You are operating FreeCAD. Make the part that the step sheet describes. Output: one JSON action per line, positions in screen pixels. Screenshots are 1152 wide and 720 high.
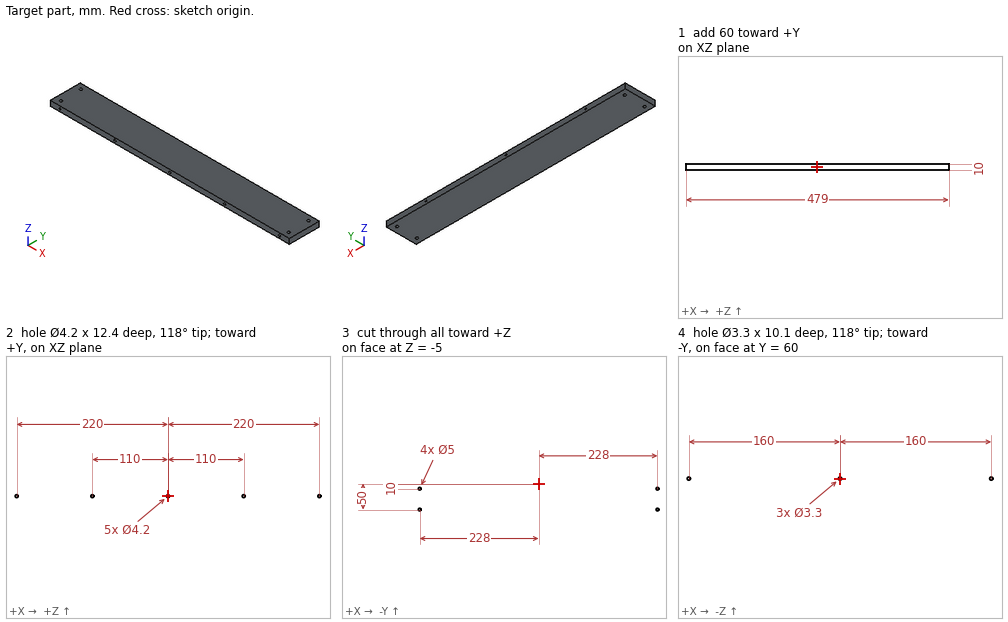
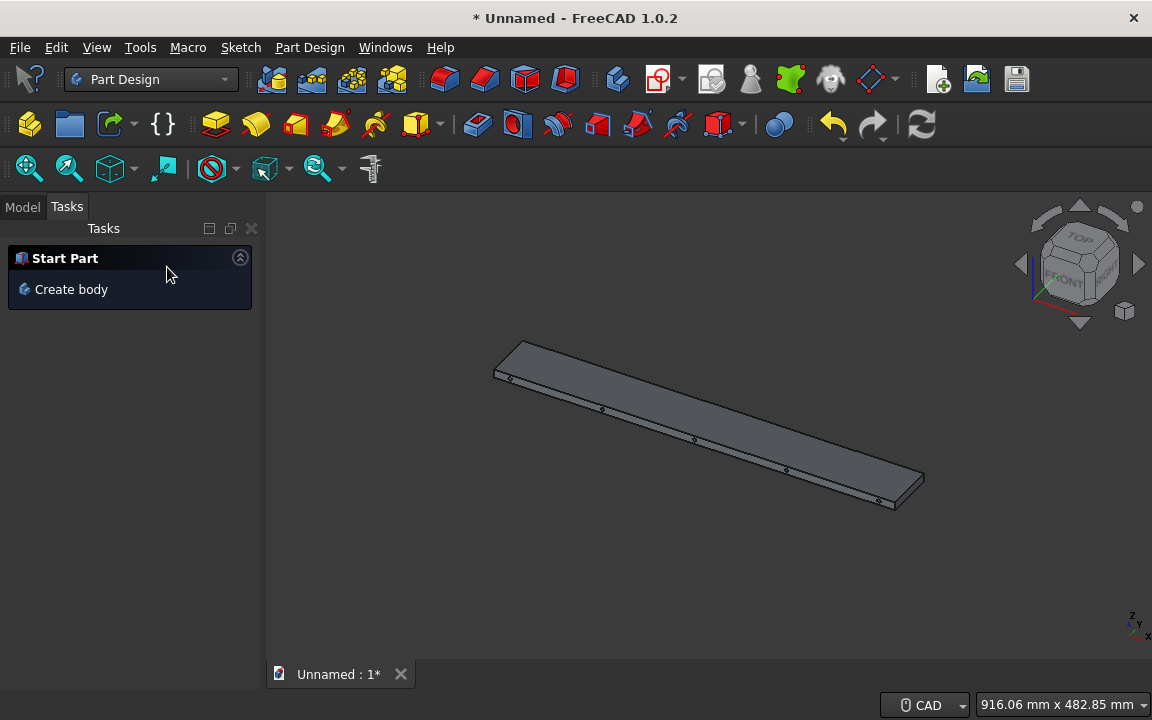
{"action": "key", "text": "5"}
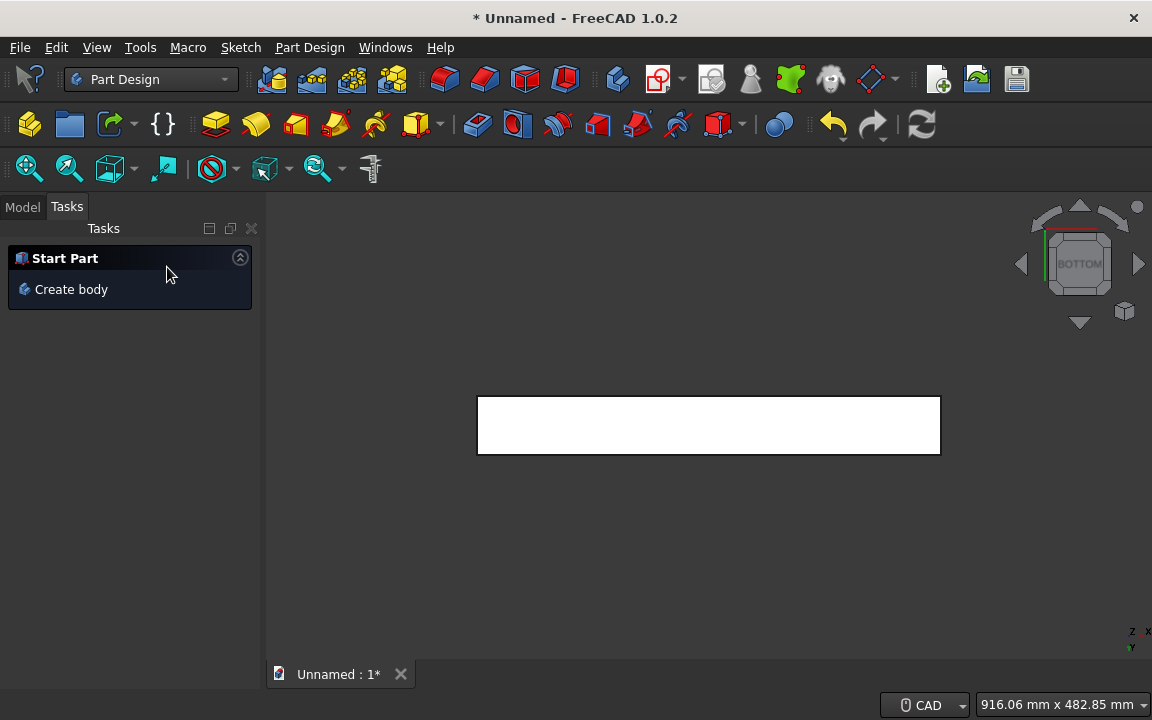
{"action": "left_click", "coordinate": [908, 425]}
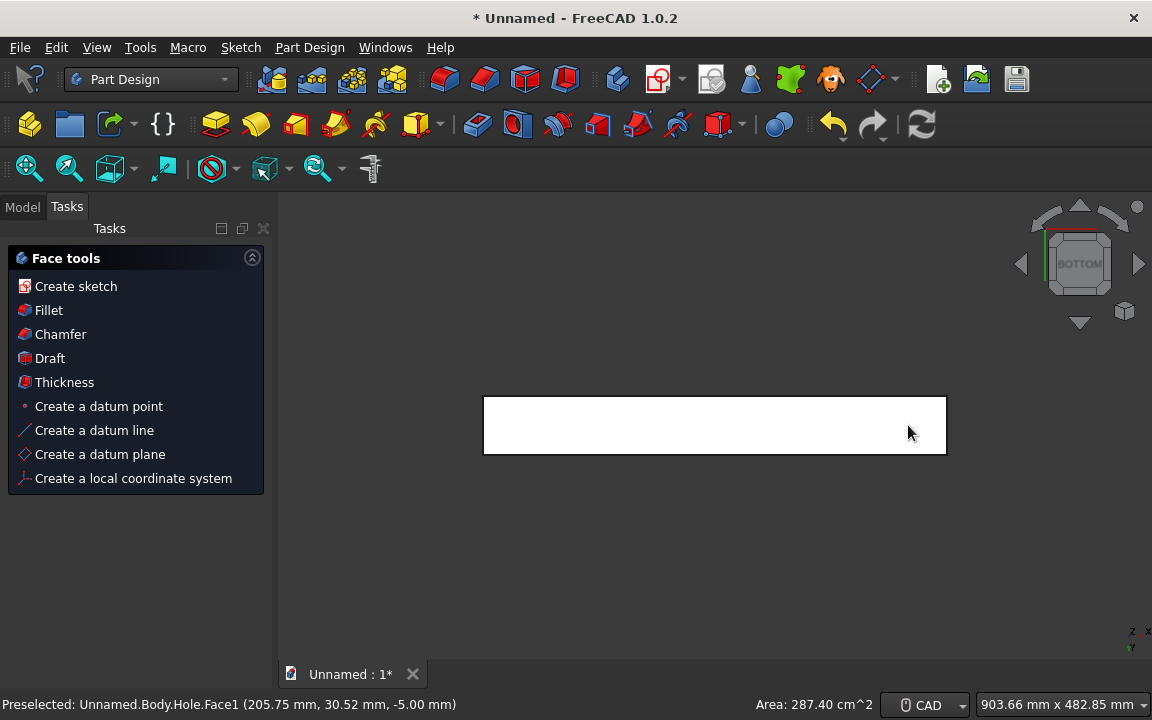
{"action": "left_click", "coordinate": [658, 80]}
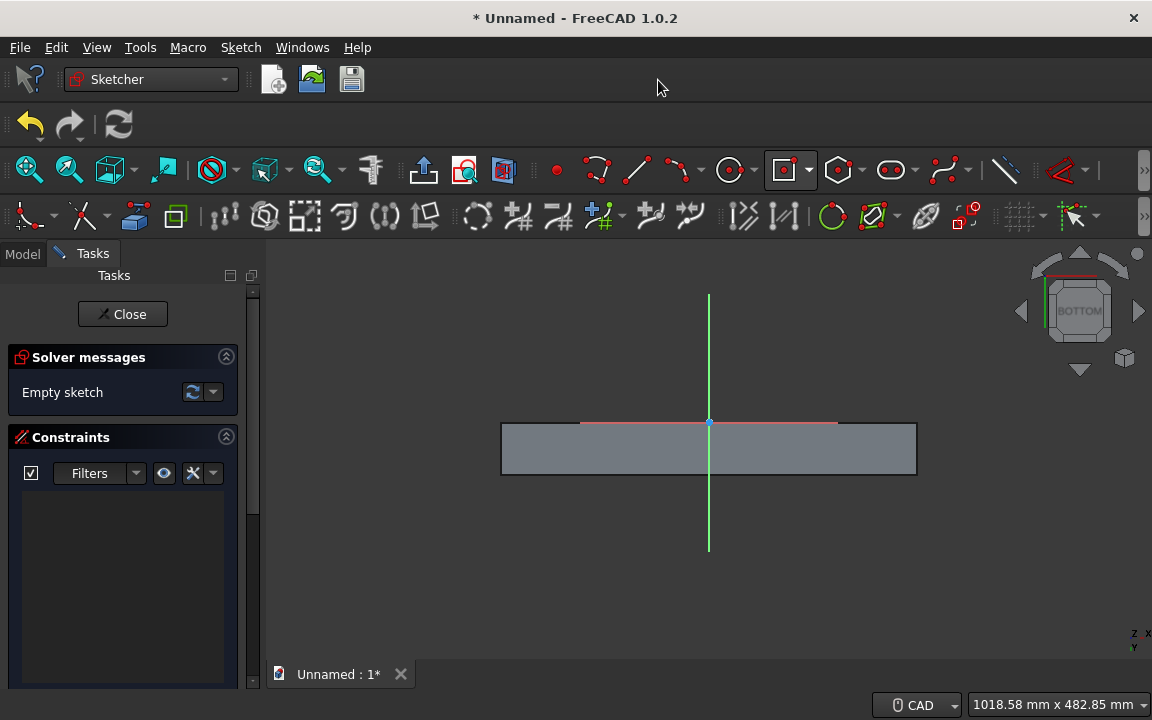
{"action": "key", "text": "g c"}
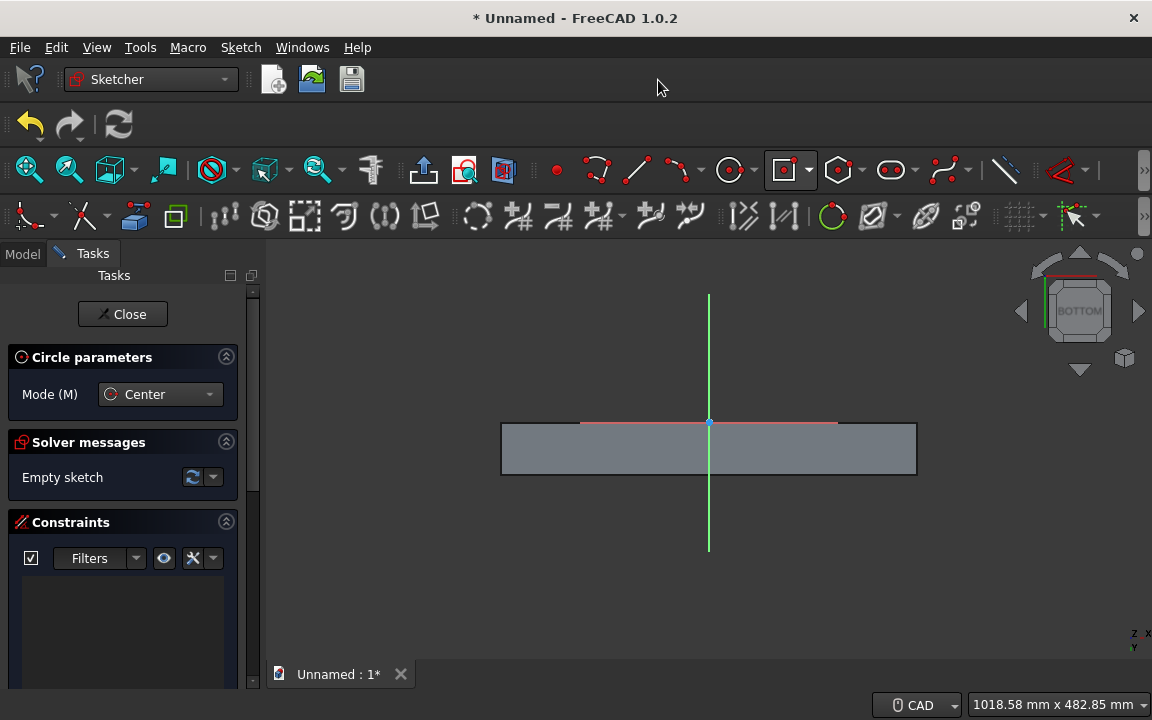
{"action": "scroll", "coordinate": [511, 466], "scroll_direction": "up", "scroll_amount": 12}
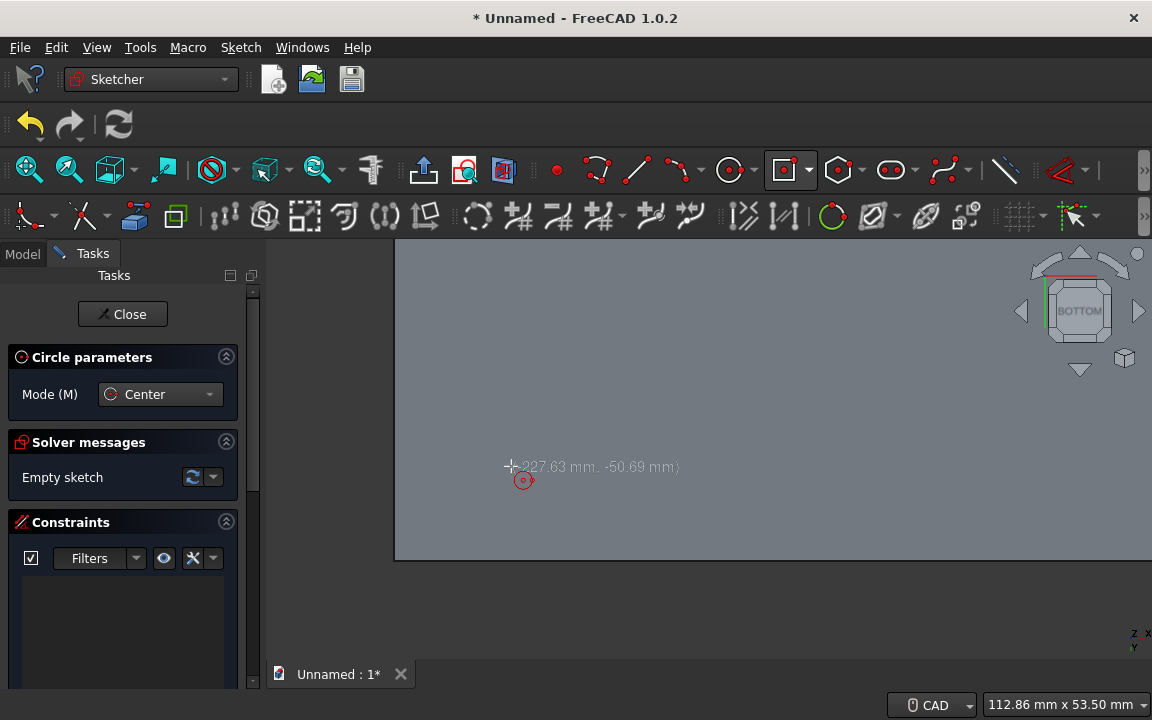
{"action": "scroll", "coordinate": [385, 475], "scroll_direction": "down", "scroll_amount": 11}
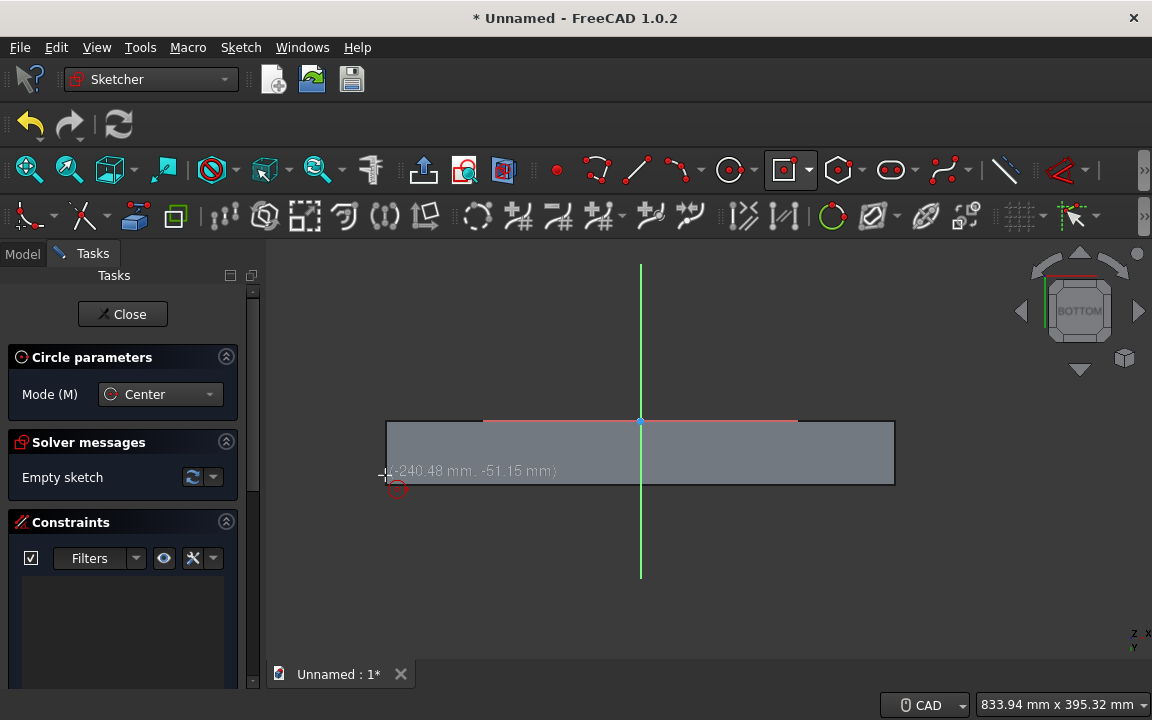
{"action": "left_click", "coordinate": [398, 474]}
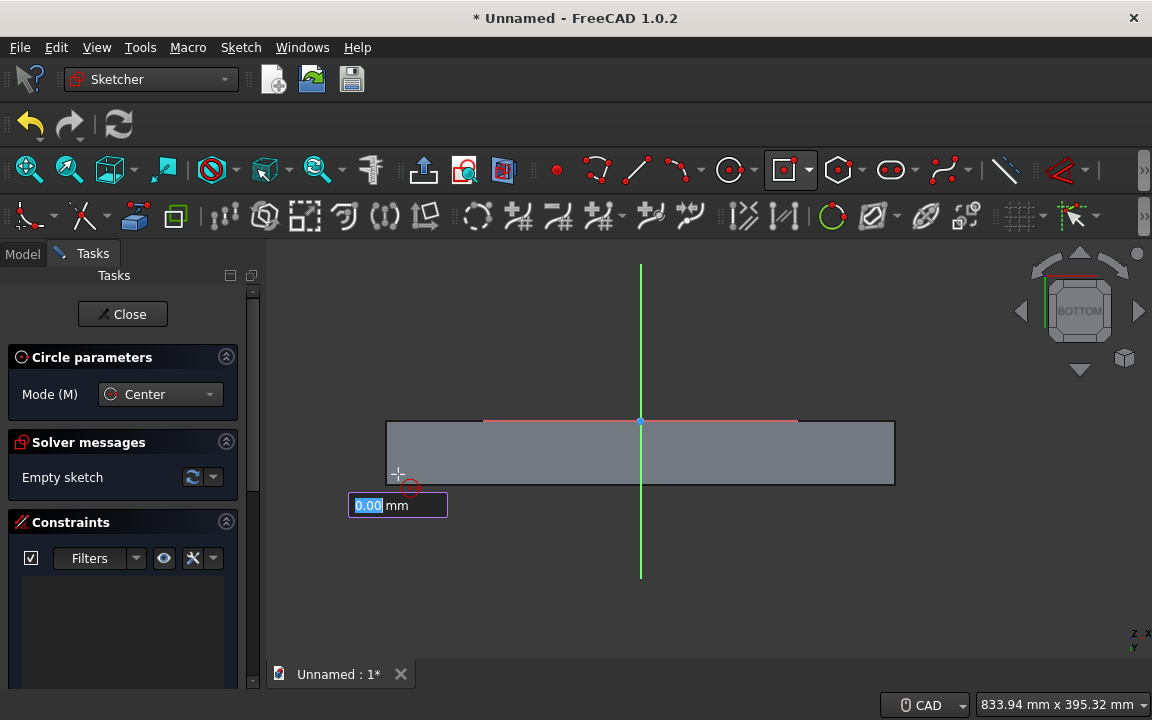
{"action": "scroll", "coordinate": [400, 473], "scroll_direction": "up", "scroll_amount": 9}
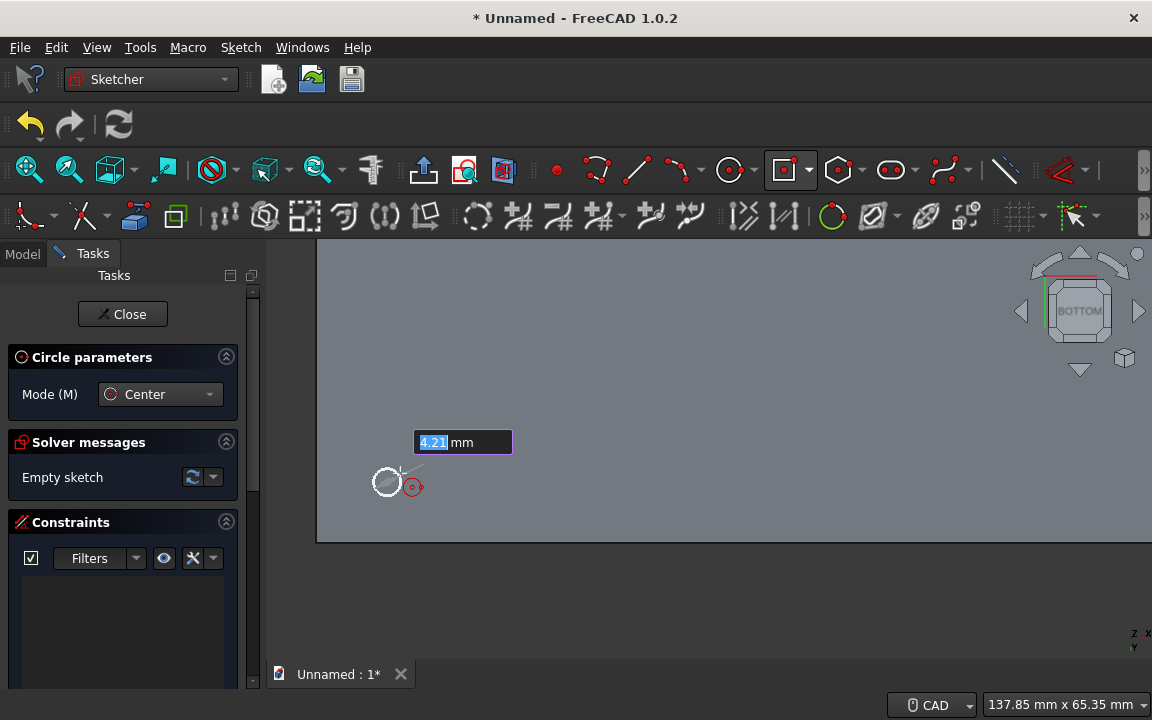
{"action": "left_click", "coordinate": [401, 467]}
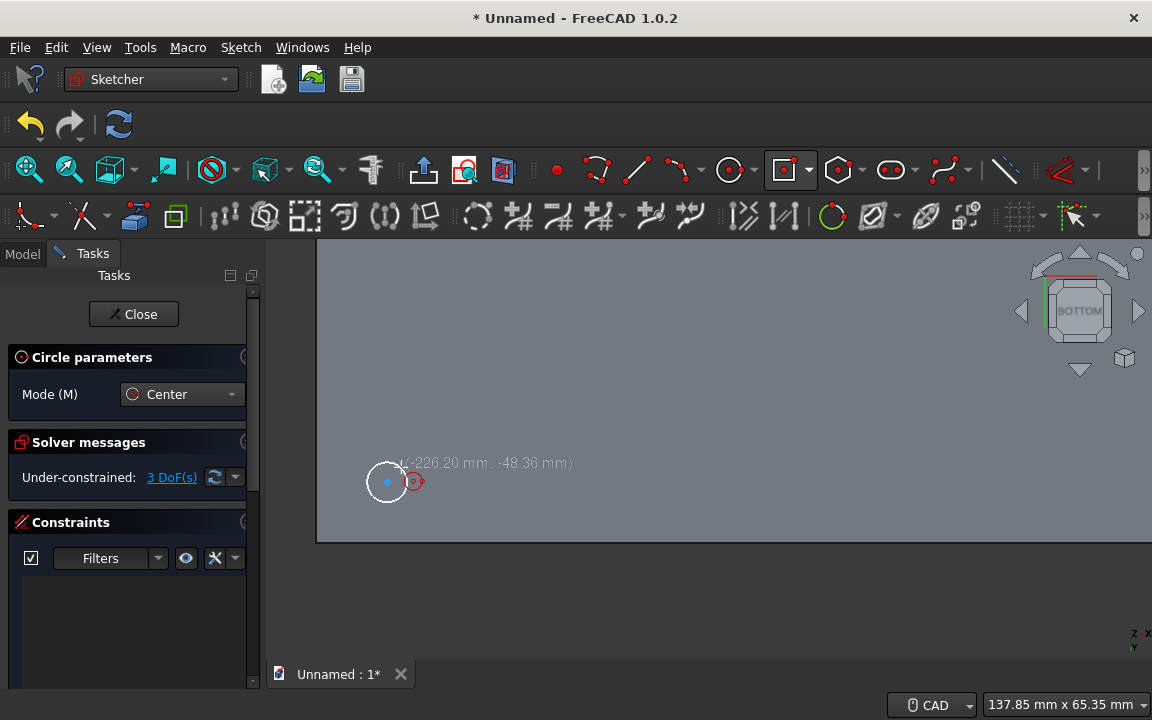
{"action": "scroll", "coordinate": [400, 473], "scroll_direction": "down", "scroll_amount": 9}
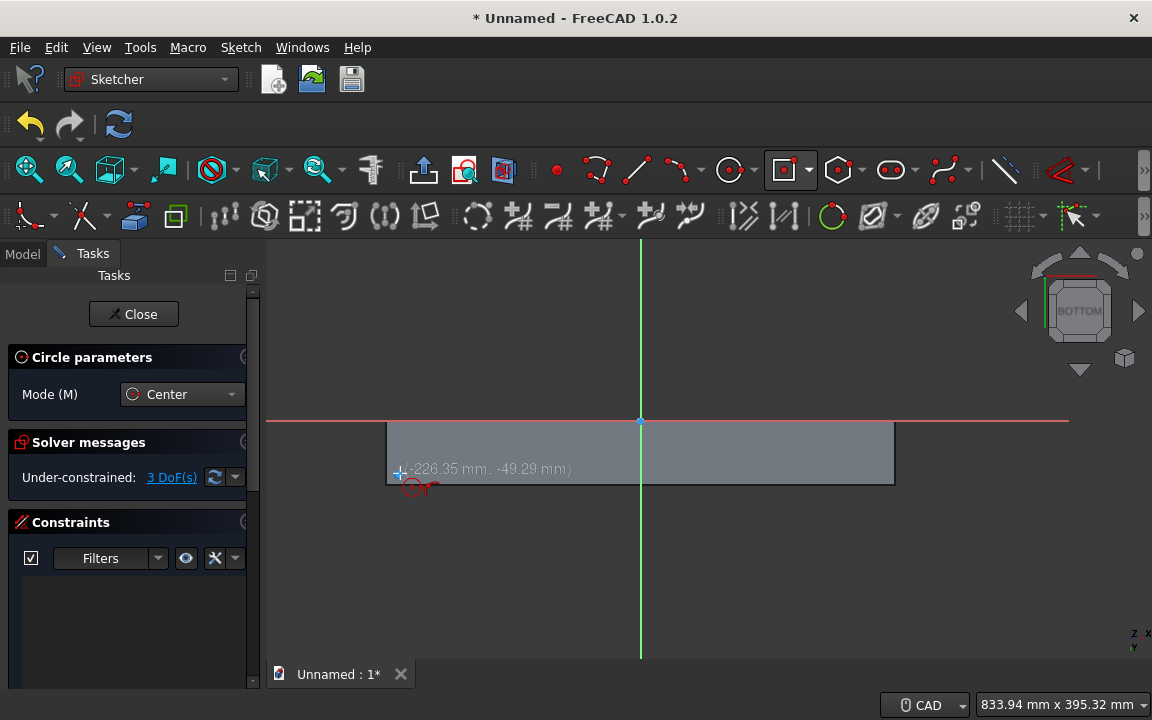
{"action": "scroll", "coordinate": [398, 432], "scroll_direction": "up", "scroll_amount": 11}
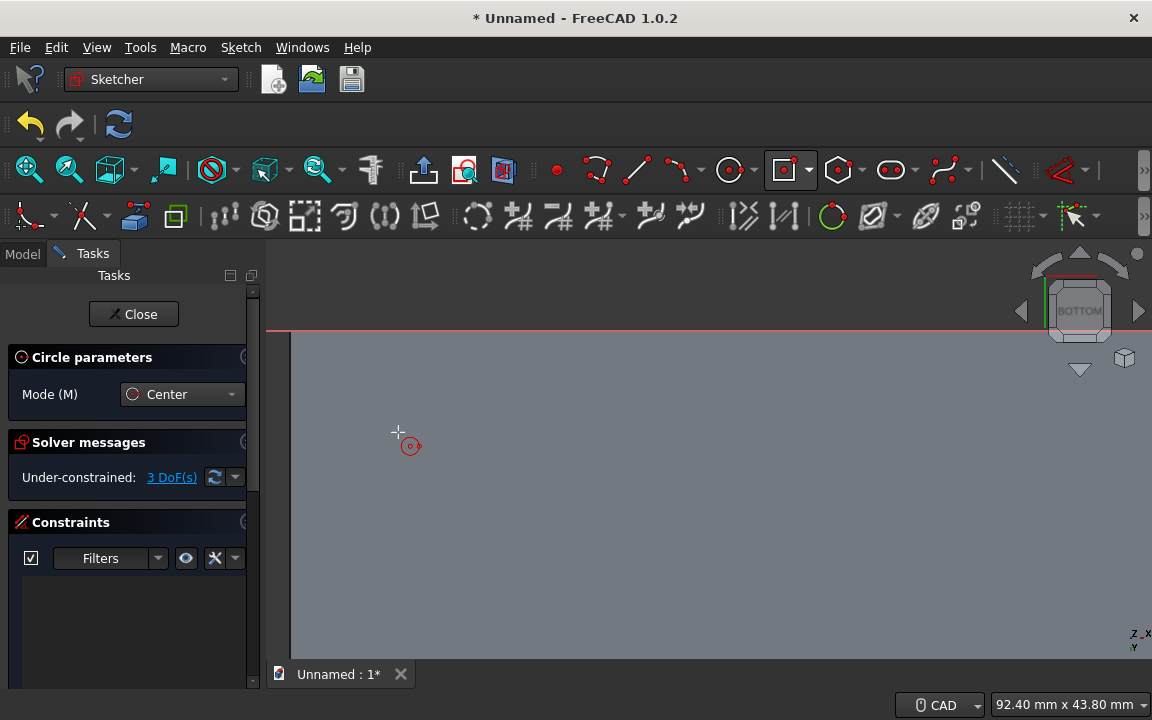
{"action": "scroll", "coordinate": [398, 432], "scroll_direction": "down", "scroll_amount": 11}